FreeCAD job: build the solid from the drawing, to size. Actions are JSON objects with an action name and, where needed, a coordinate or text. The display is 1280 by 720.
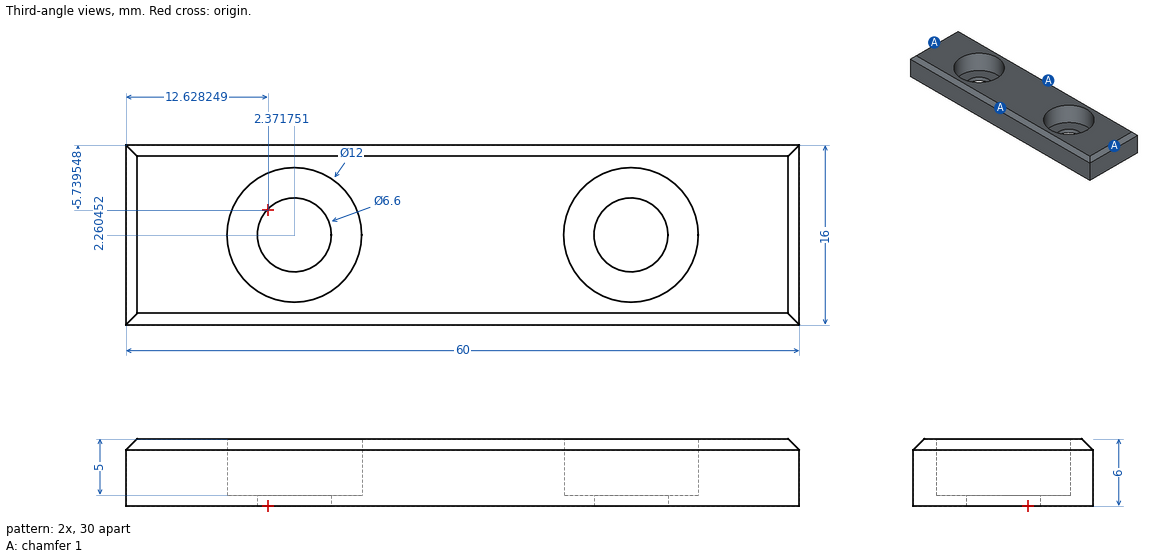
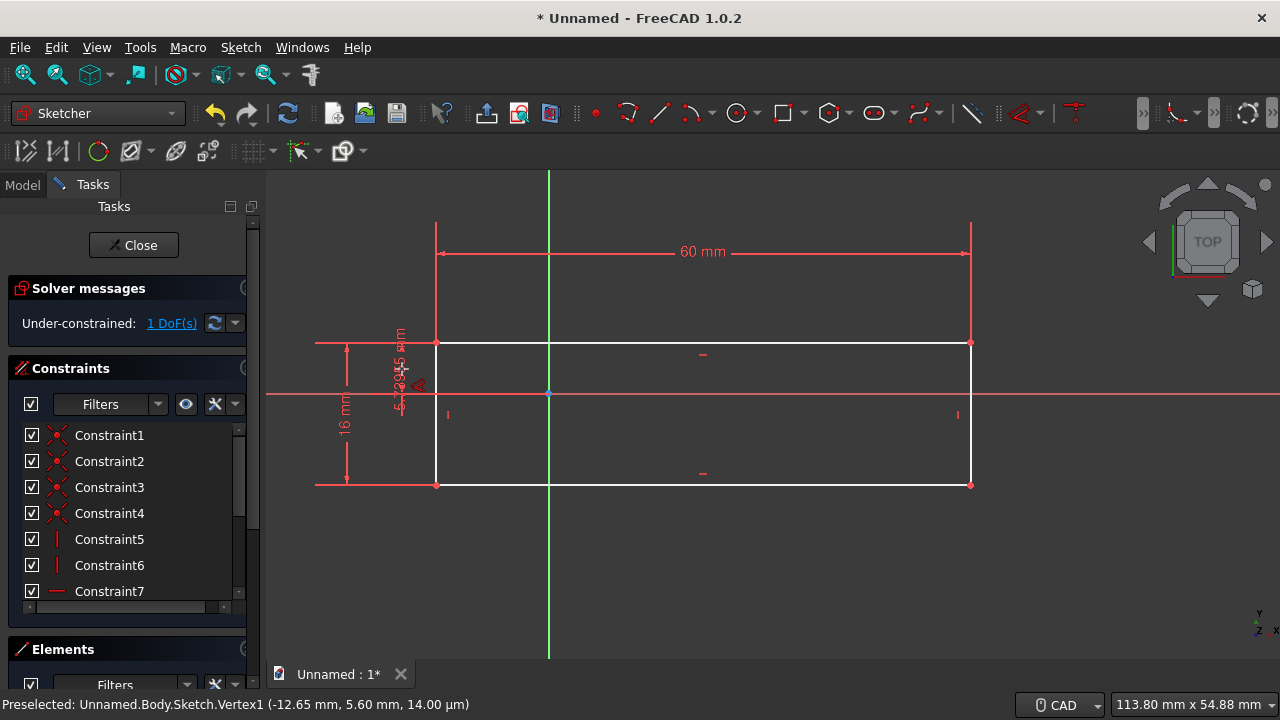
{"action": "left_click", "coordinate": [436, 343]}
{"action": "left_click", "coordinate": [492, 309]}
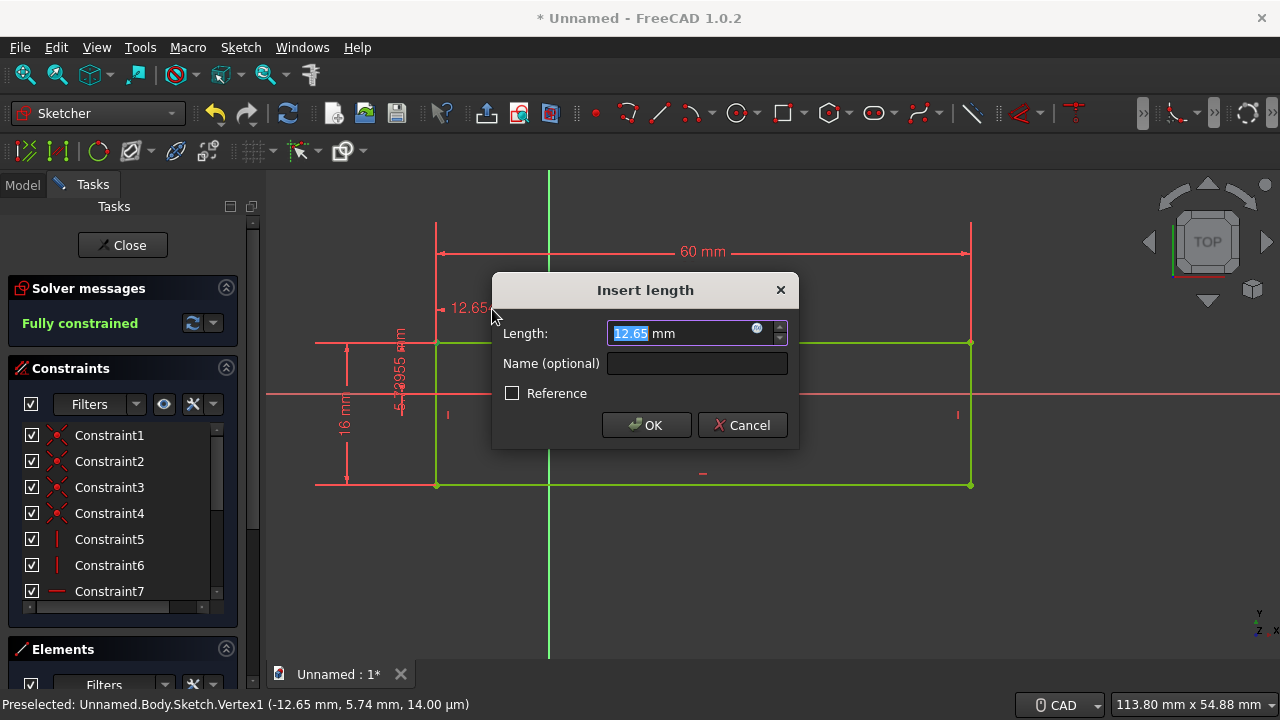
{"action": "type", "text": "12.628249"}
{"action": "key", "text": "Return"}
{"action": "key", "text": "Escape"}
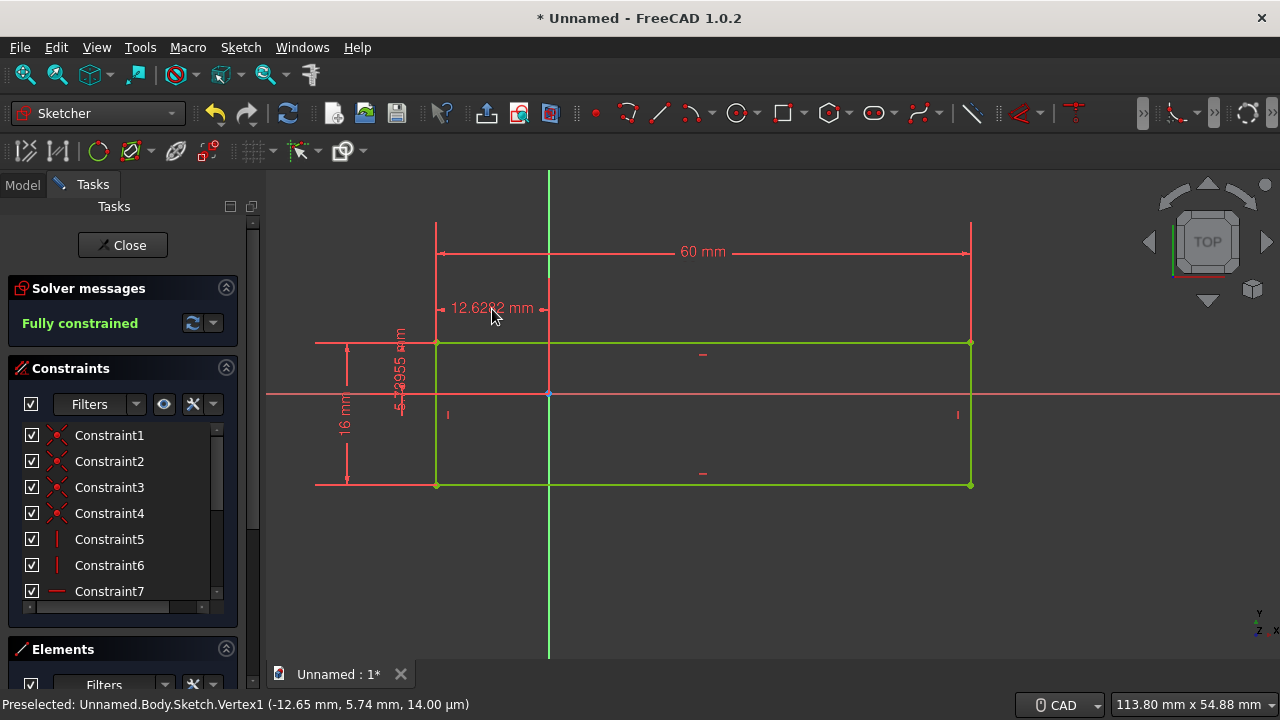
{"action": "left_click", "coordinate": [123, 245]}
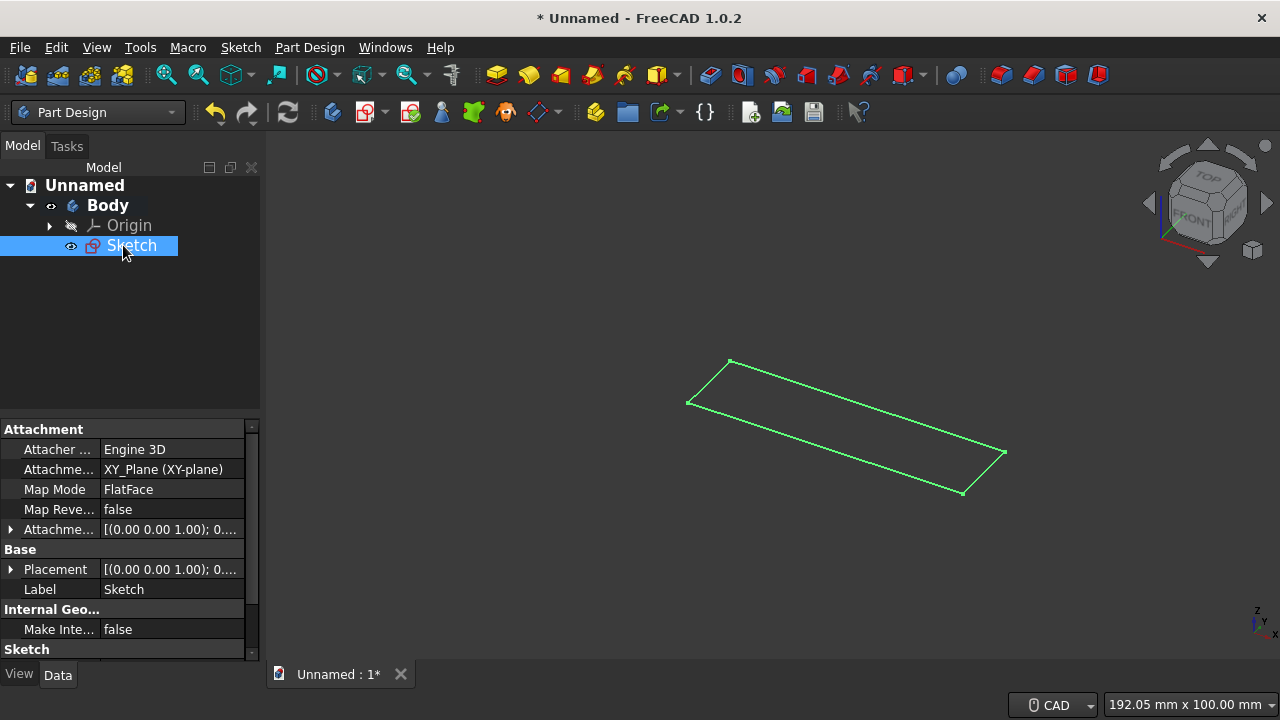
{"action": "left_click", "coordinate": [498, 76]}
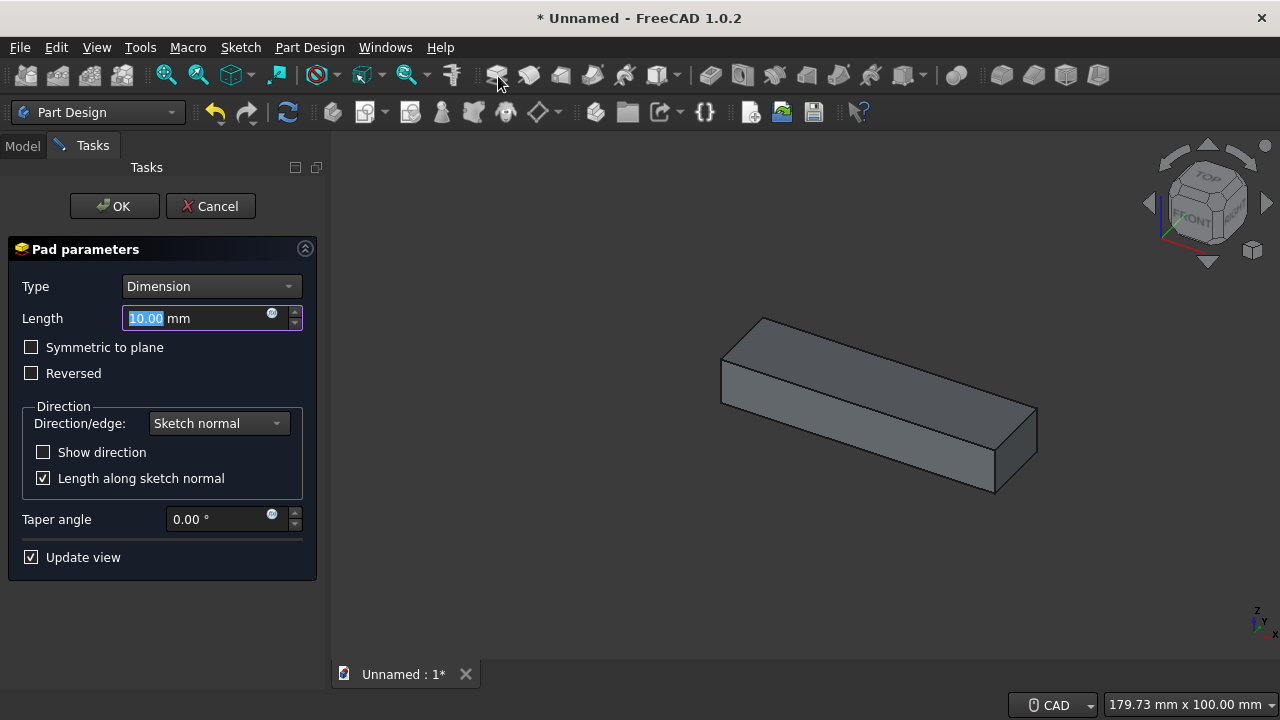
{"action": "type", "text": "6"}
{"action": "key", "text": "Tab"}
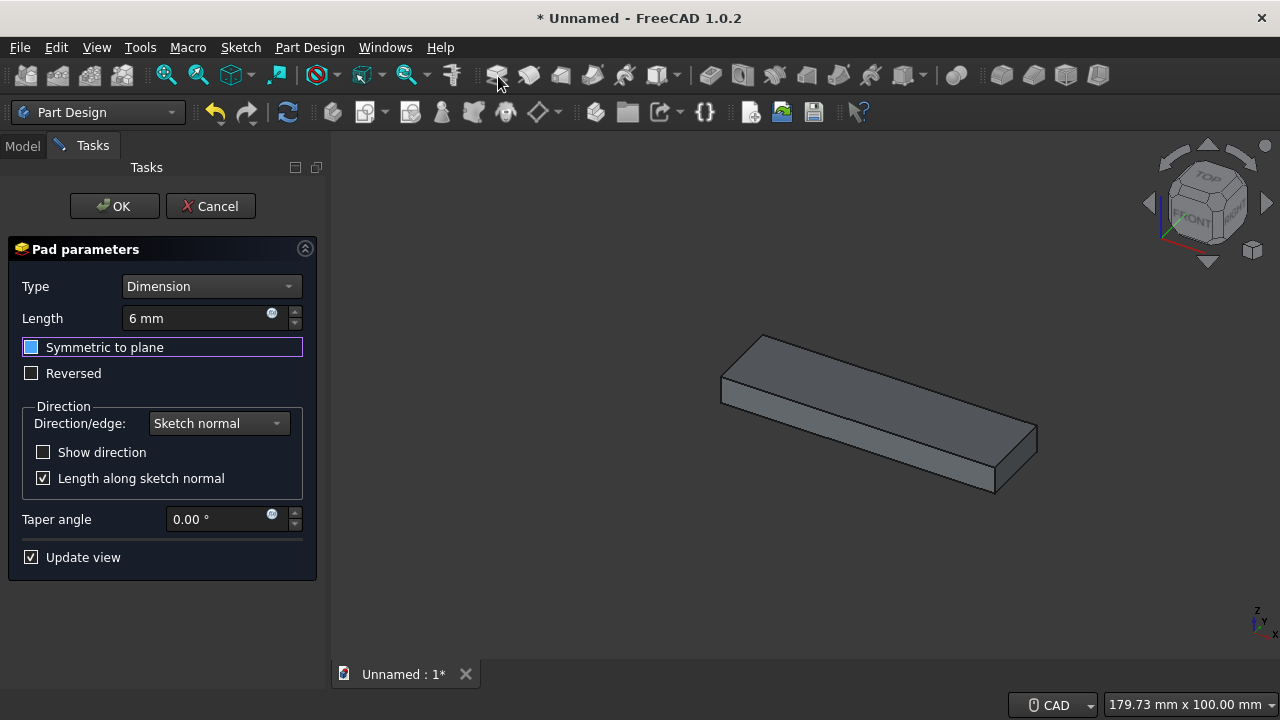
{"action": "left_click", "coordinate": [115, 206]}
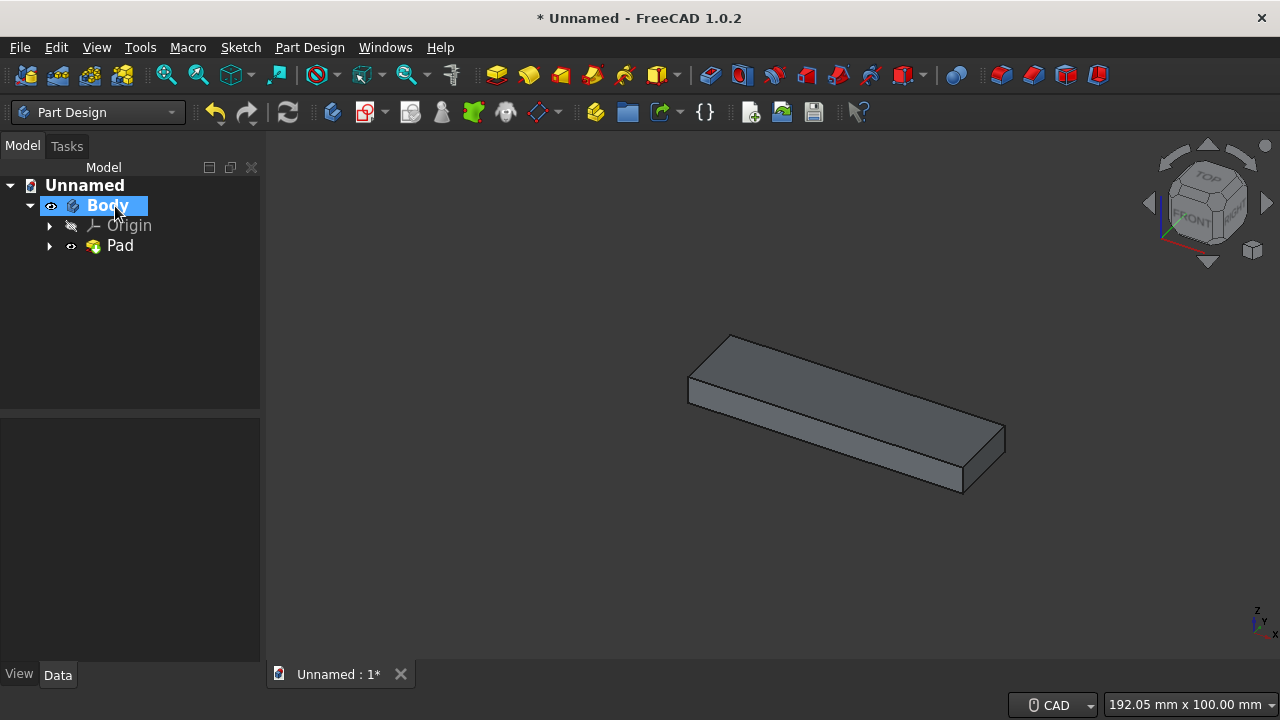
{"action": "left_click", "coordinate": [168, 76]}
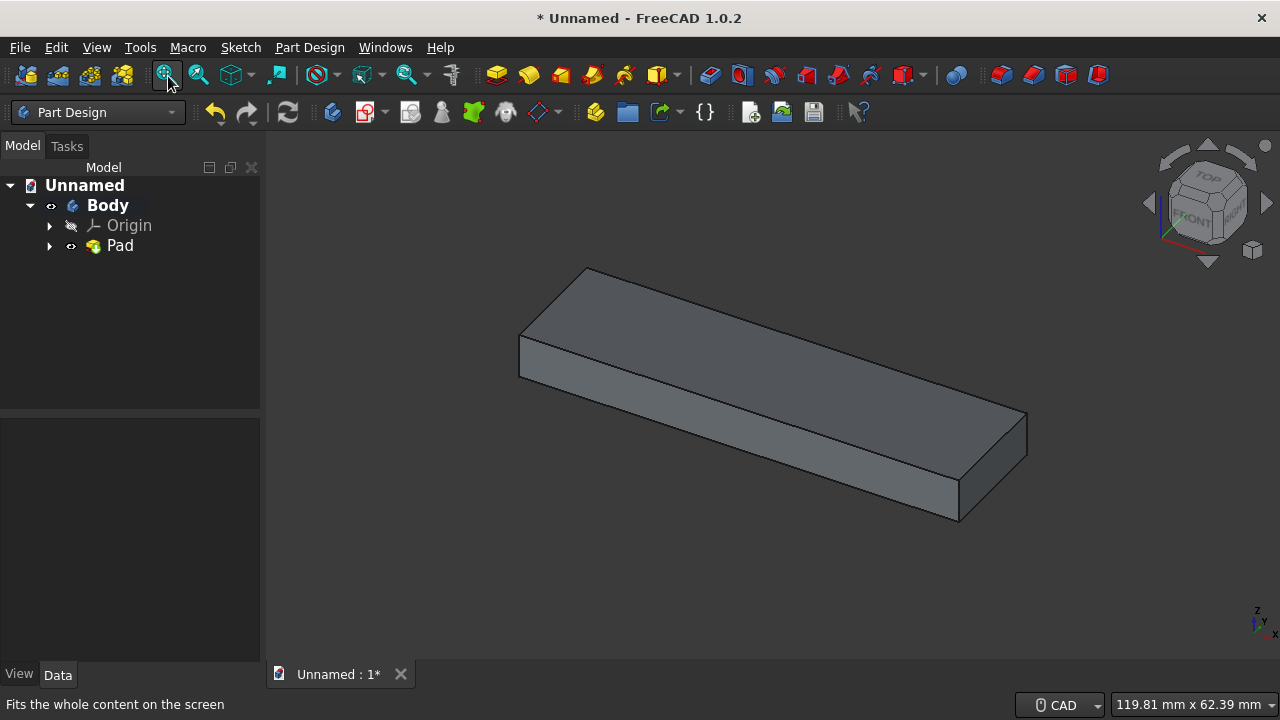
{"action": "left_click", "coordinate": [899, 415]}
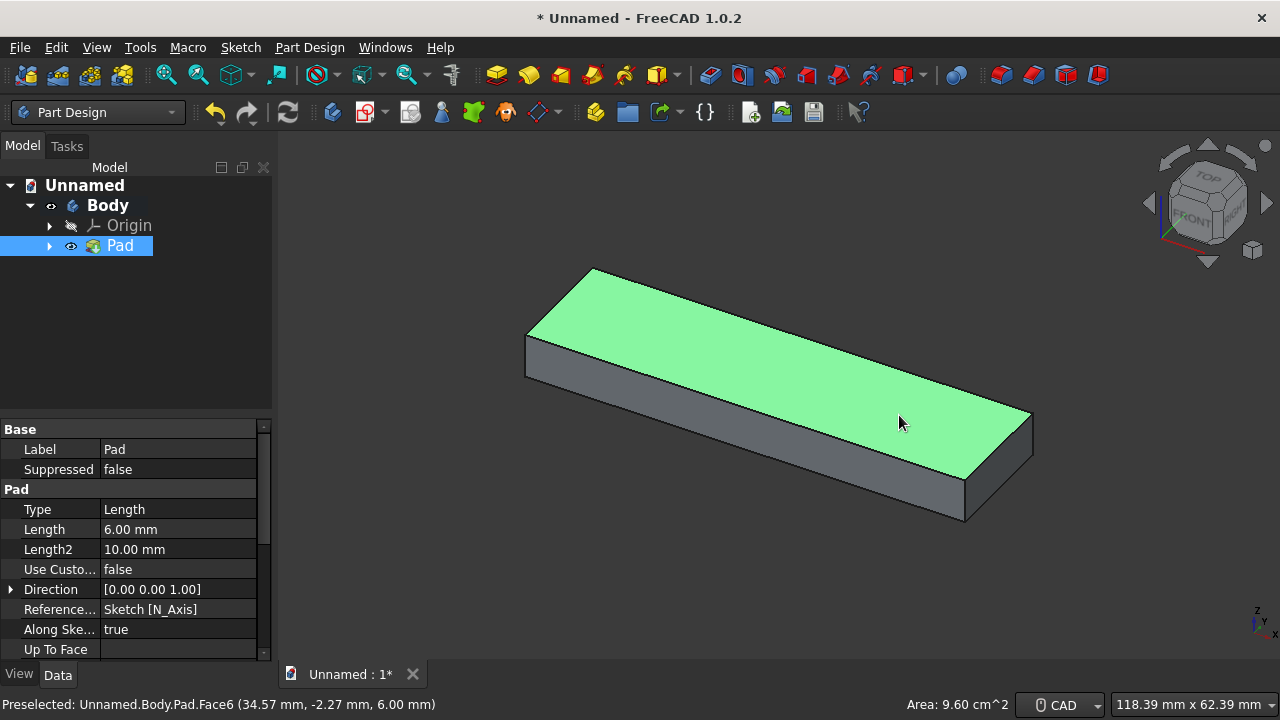
{"action": "left_click", "coordinate": [366, 112]}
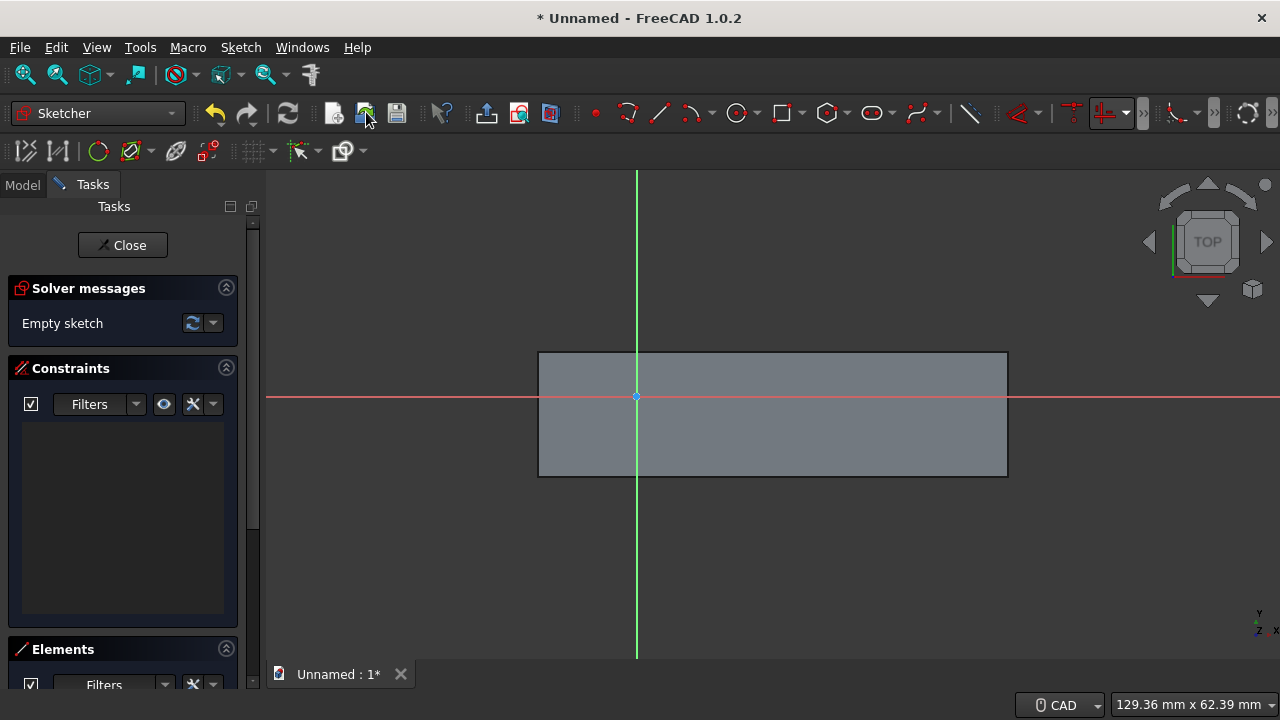
{"action": "scroll", "coordinate": [646, 414], "scroll_direction": "up", "scroll_amount": 9}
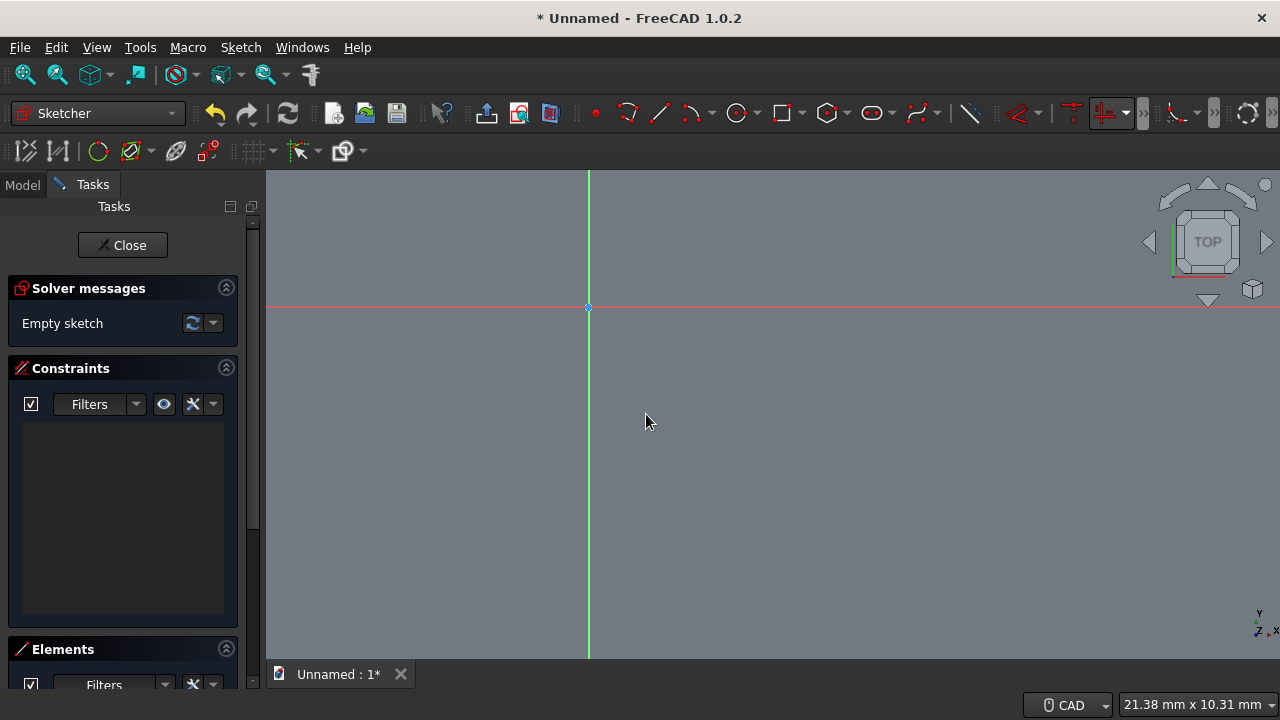
{"action": "left_click", "coordinate": [738, 114]}